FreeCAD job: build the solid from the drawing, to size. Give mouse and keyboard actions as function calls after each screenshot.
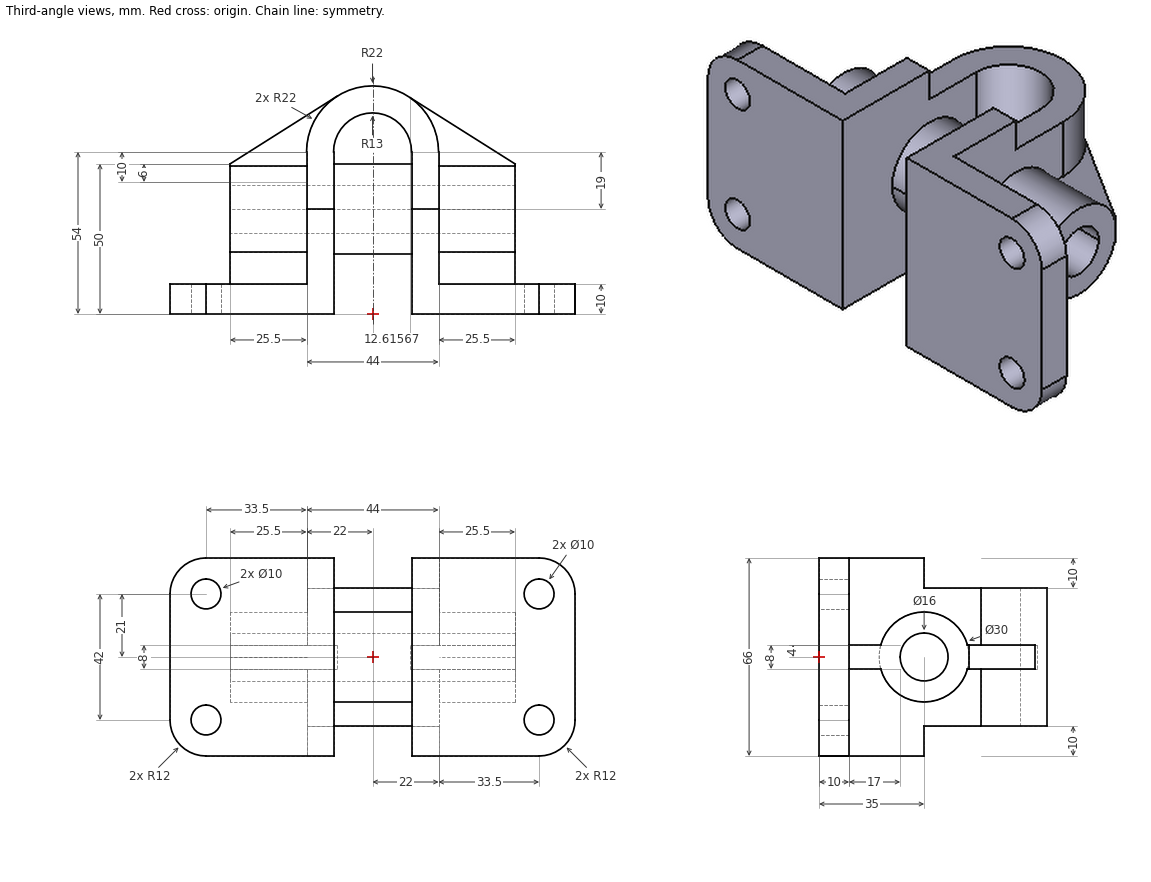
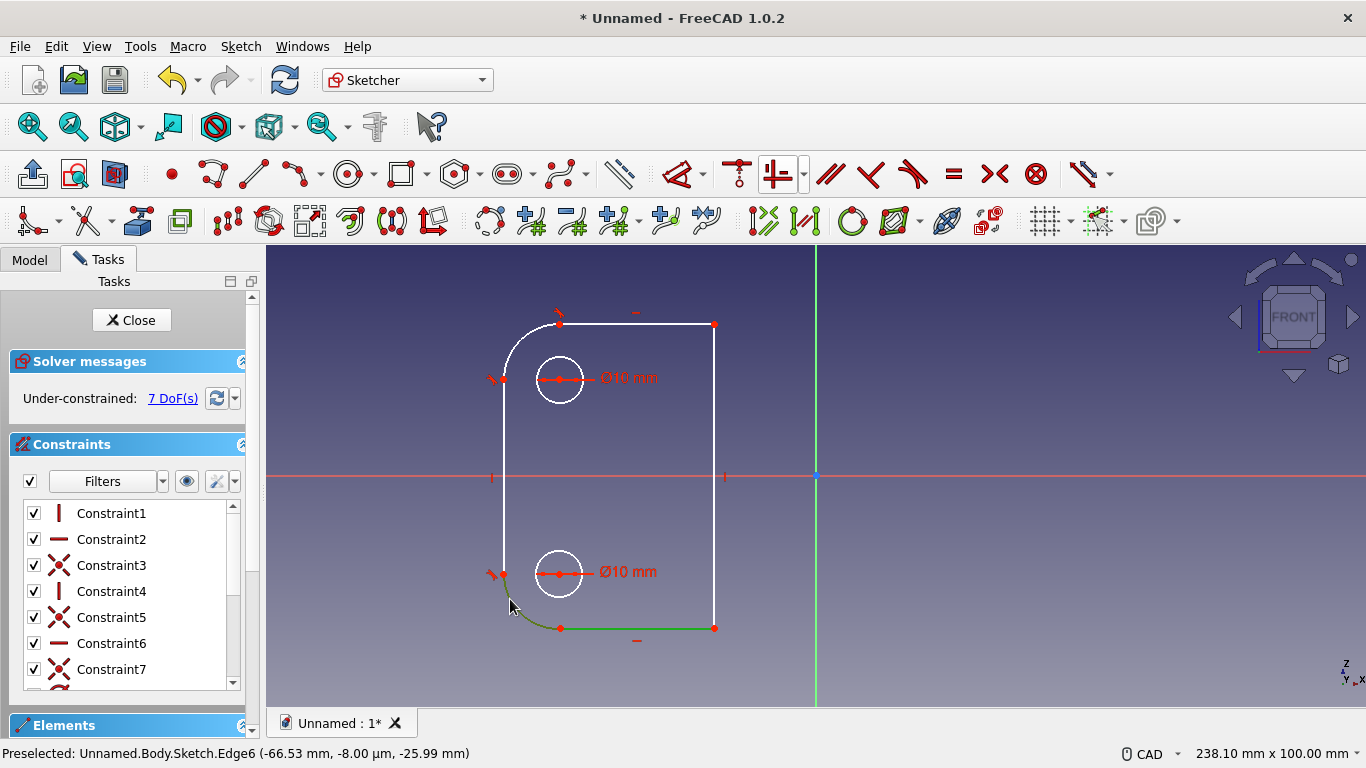
click(913, 174)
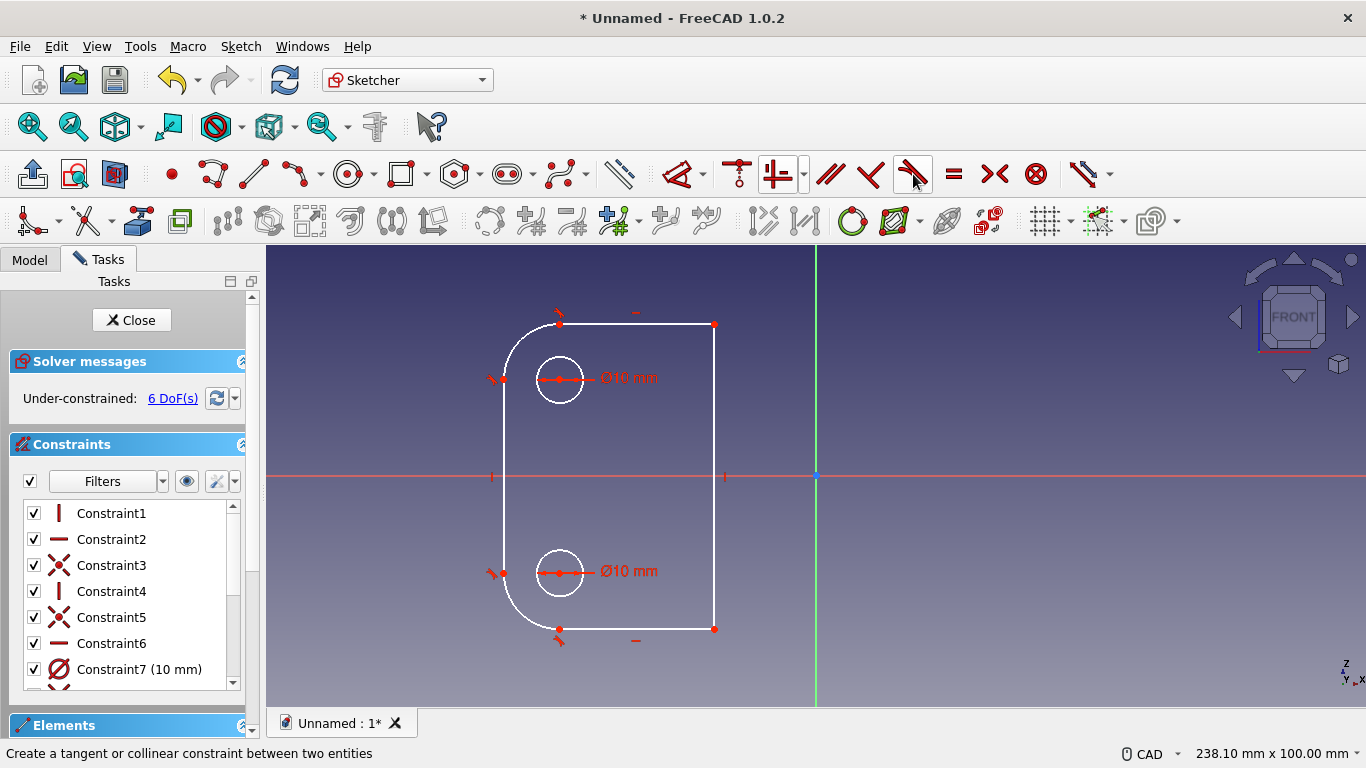
click(535, 330)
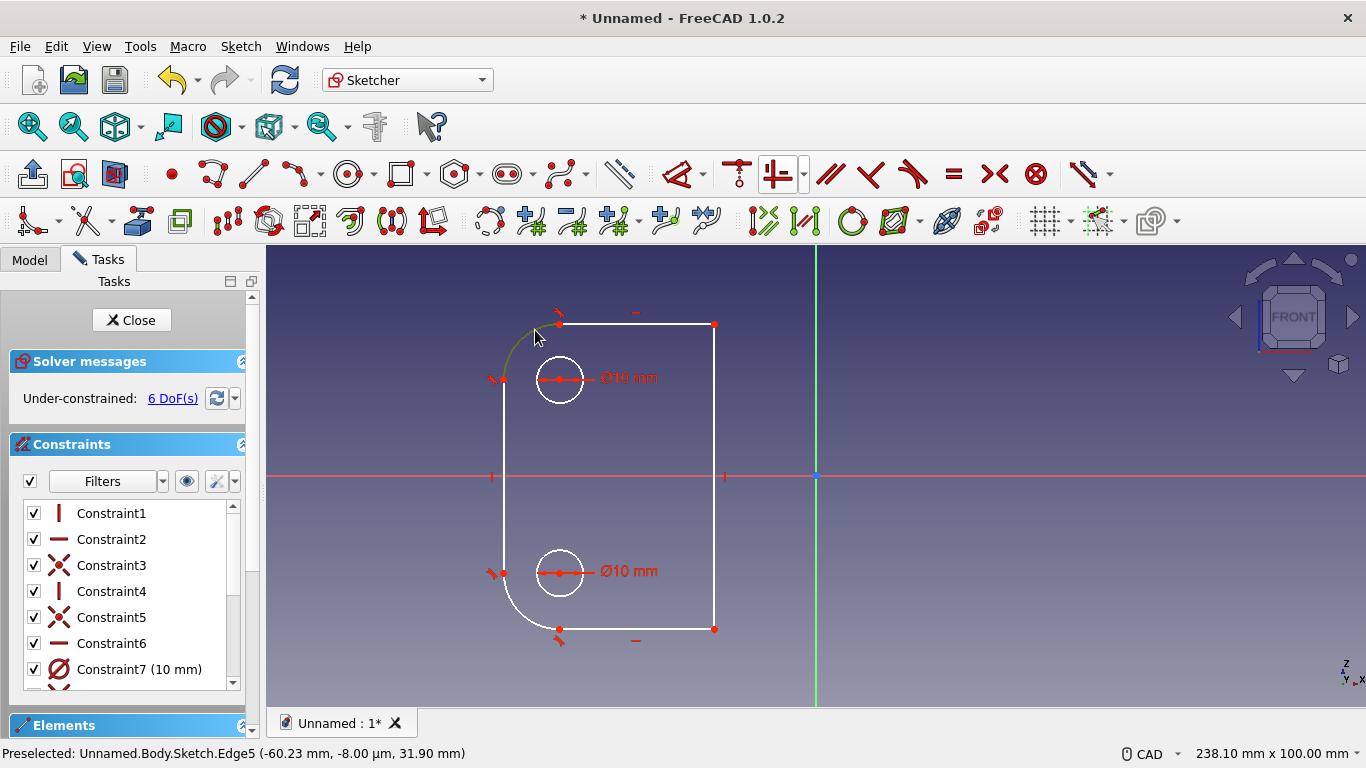
click(510, 599)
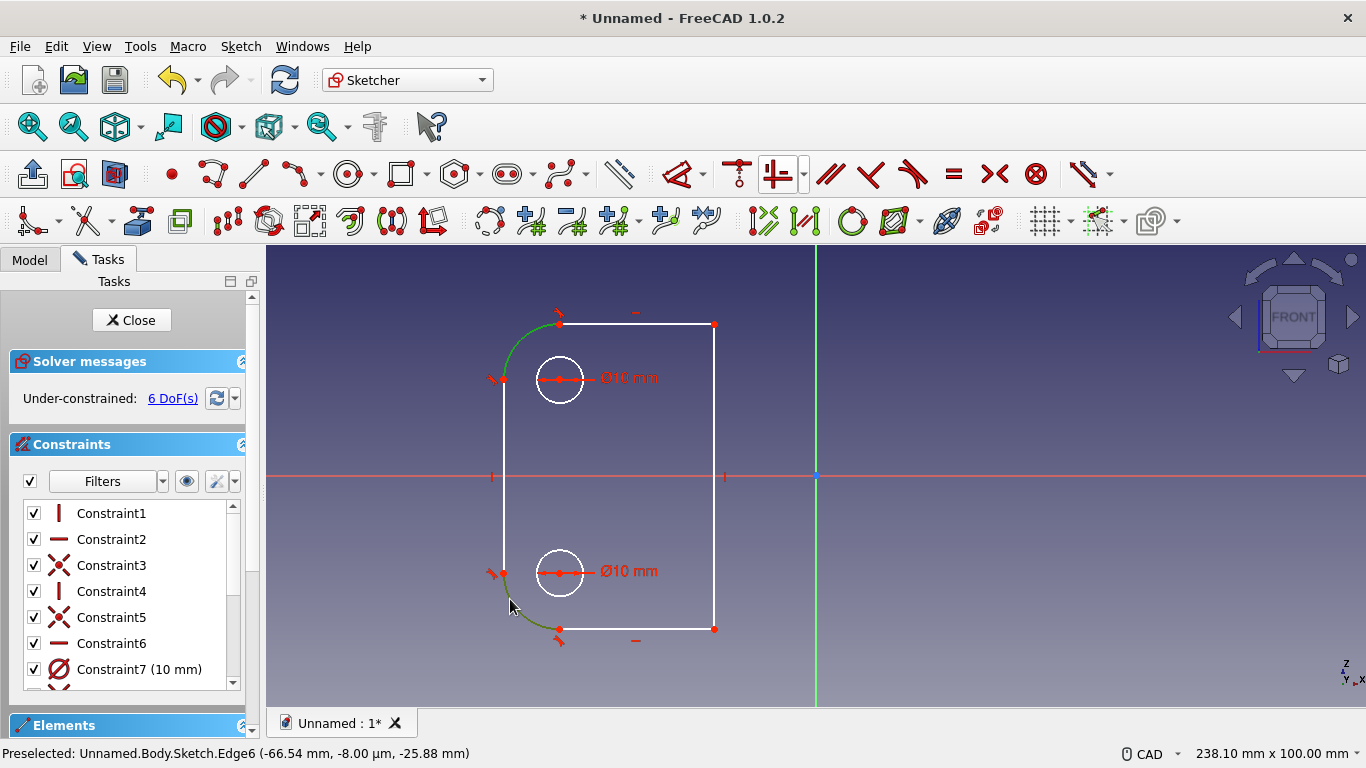
click(954, 174)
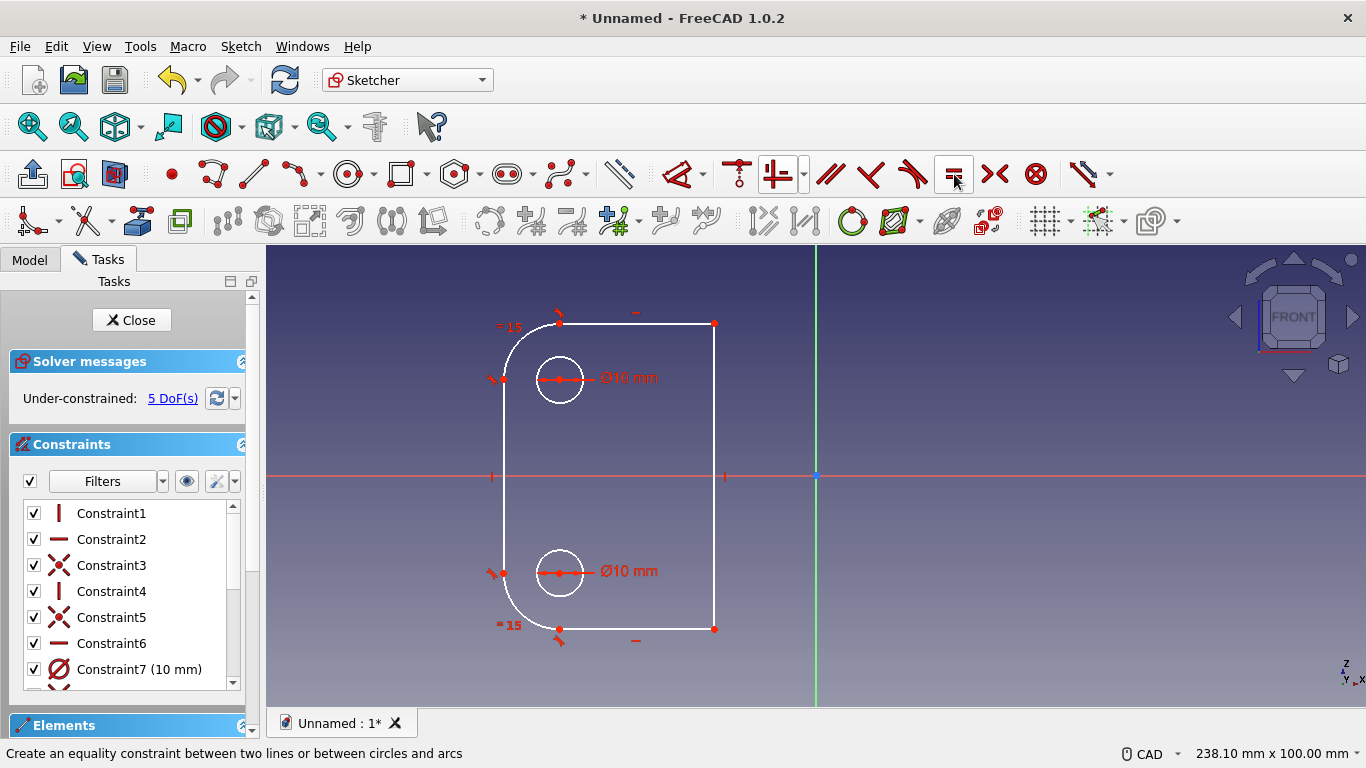
click(535, 330)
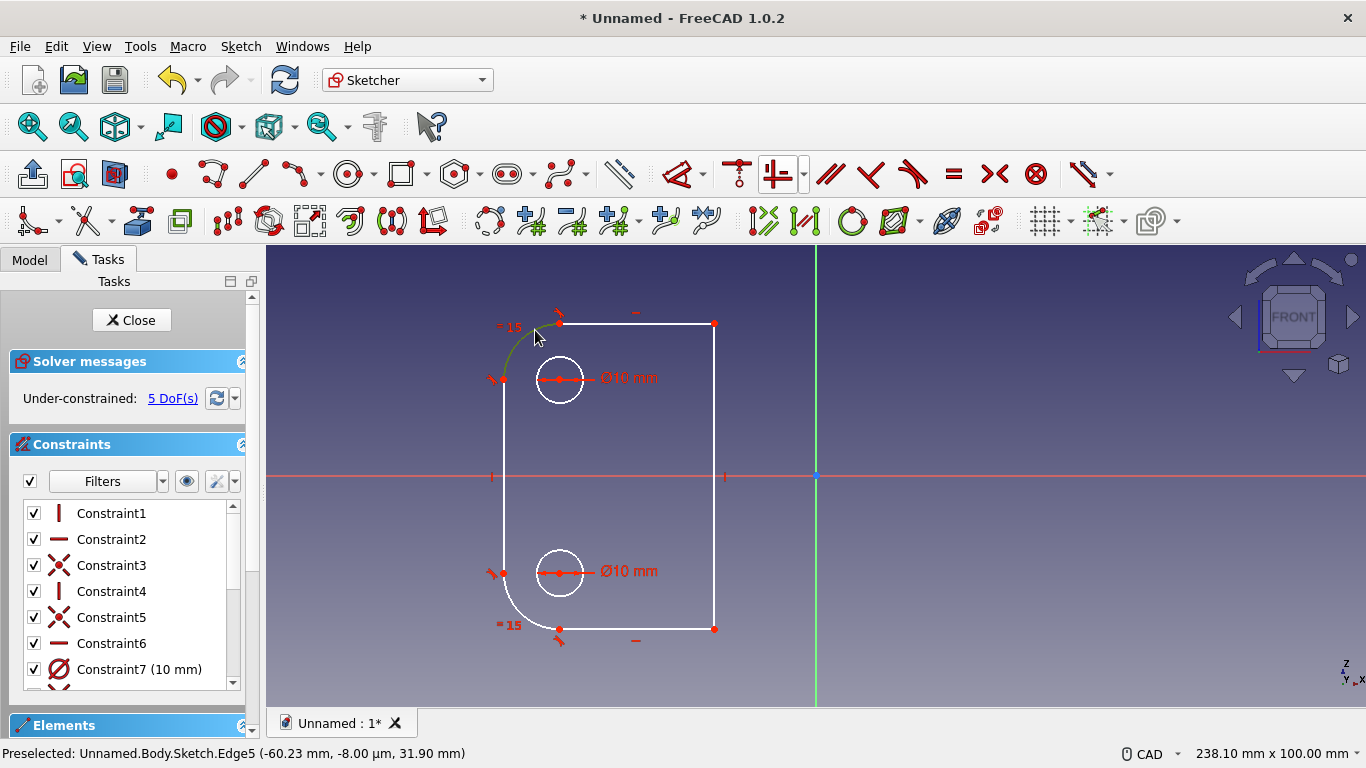
click(702, 174)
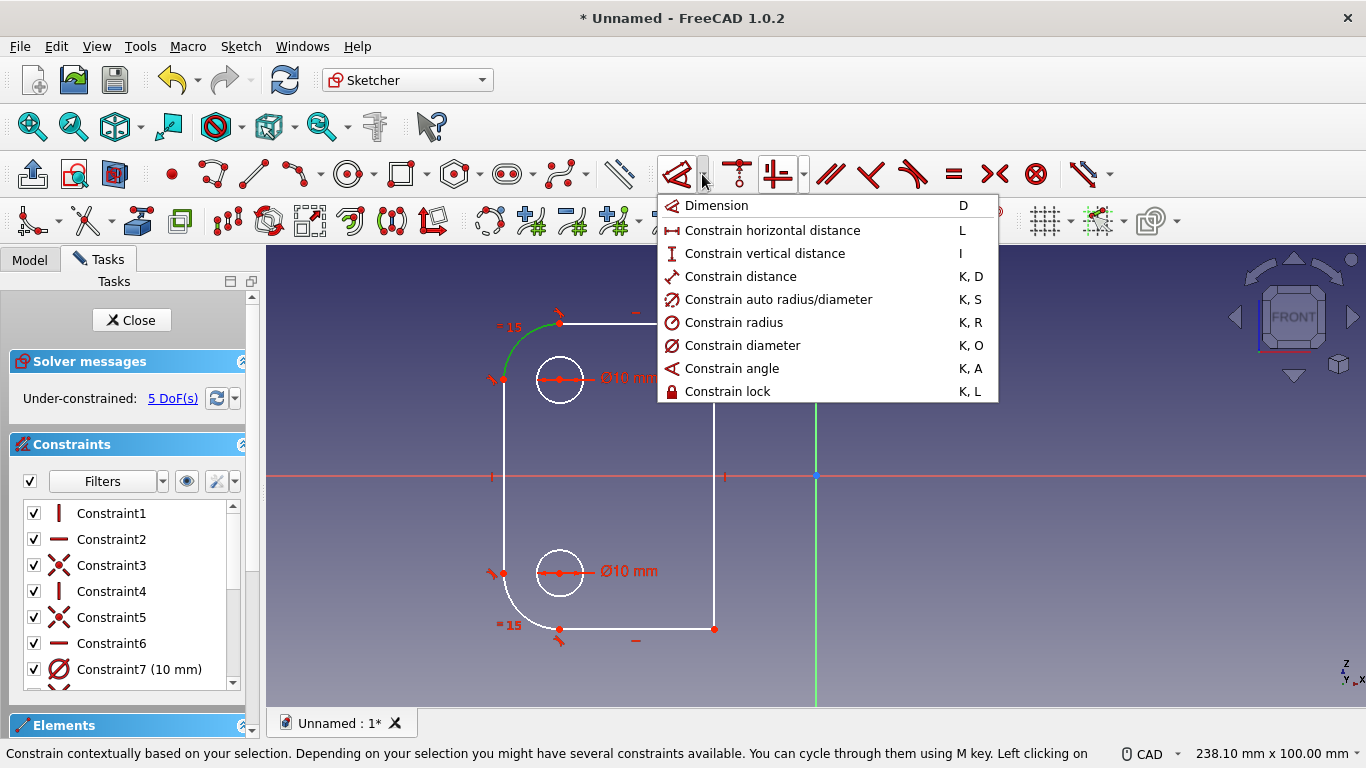
click(828, 322)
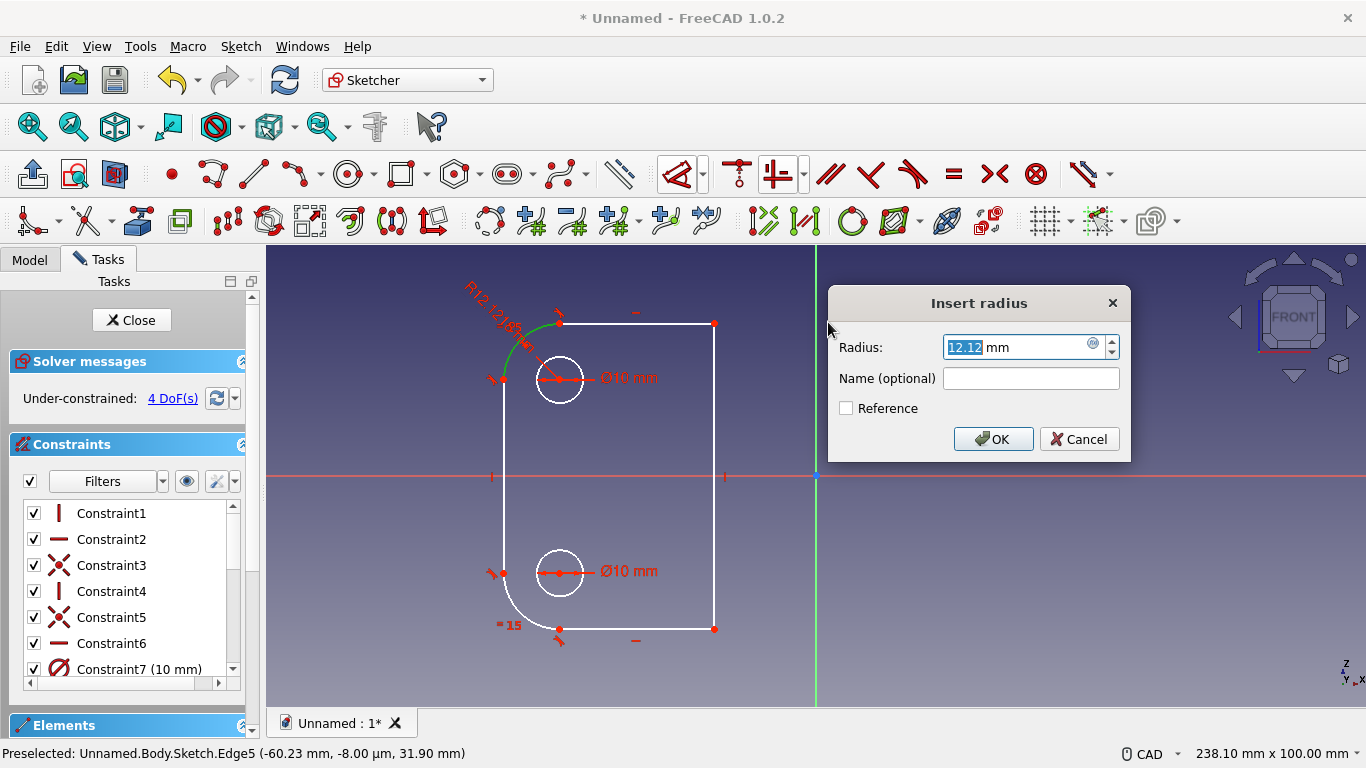
text(12)
key(Return)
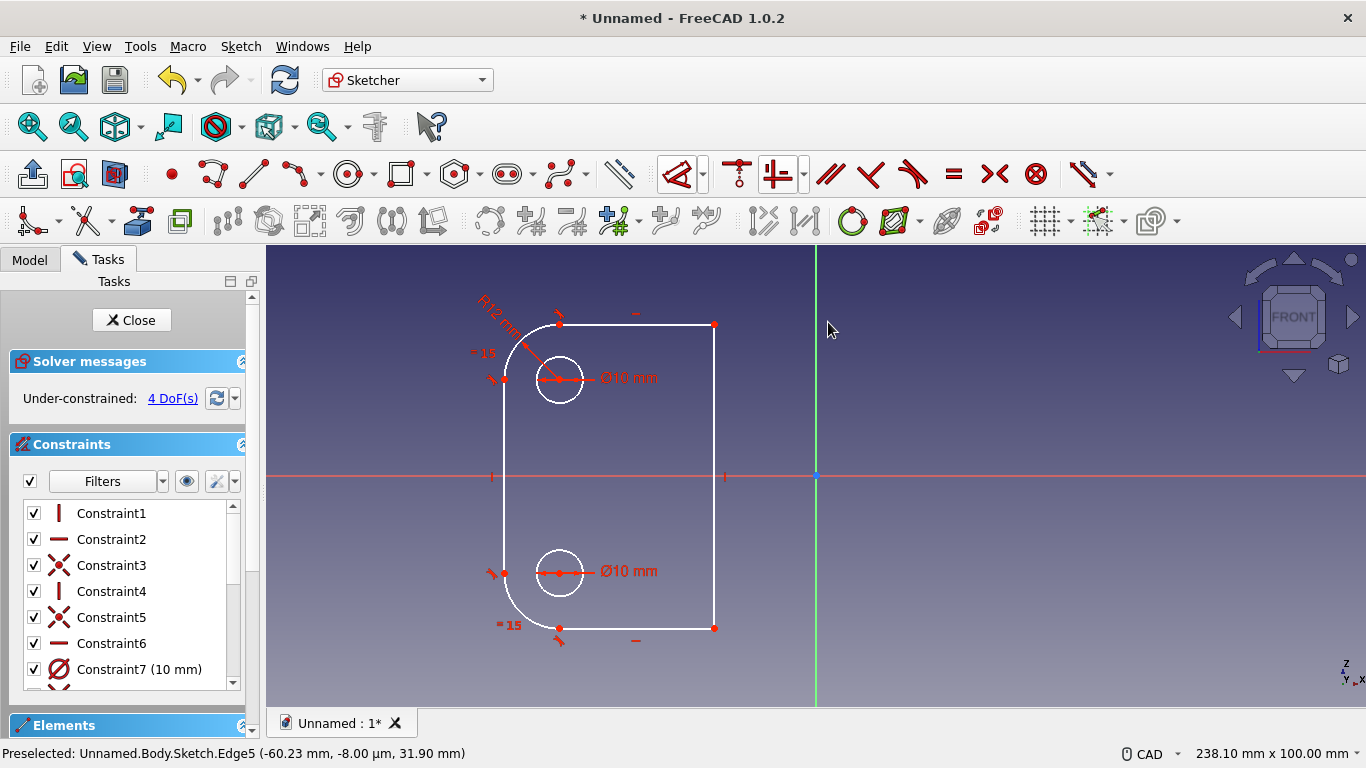
click(504, 515)